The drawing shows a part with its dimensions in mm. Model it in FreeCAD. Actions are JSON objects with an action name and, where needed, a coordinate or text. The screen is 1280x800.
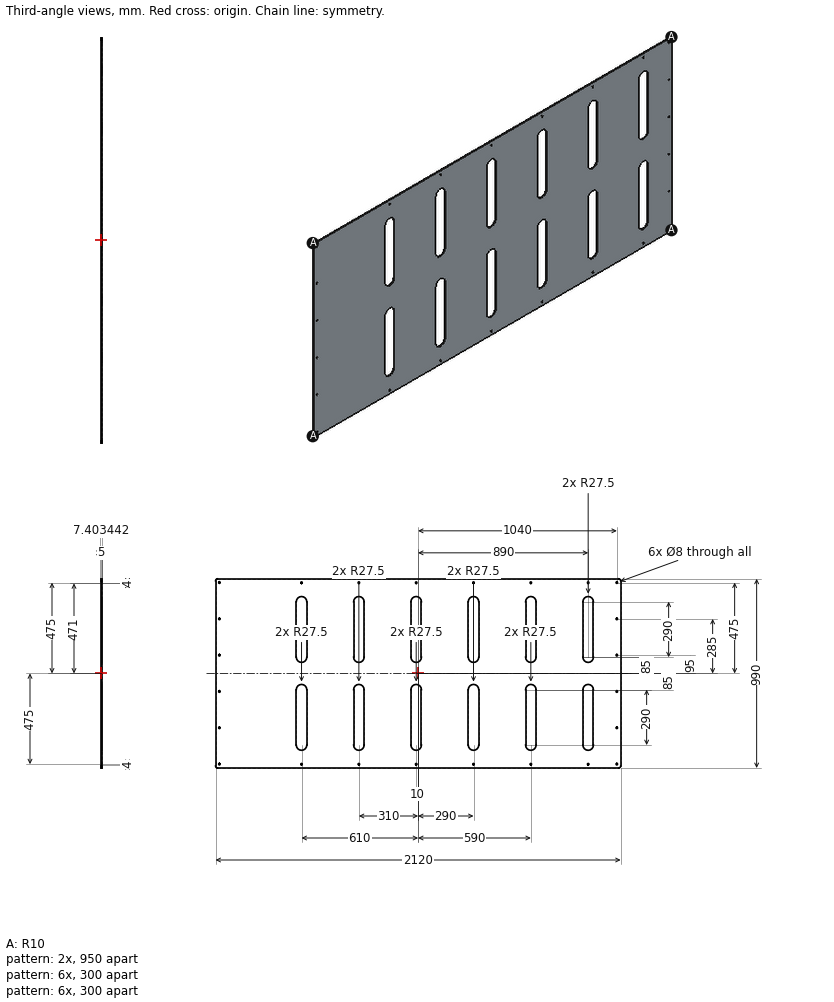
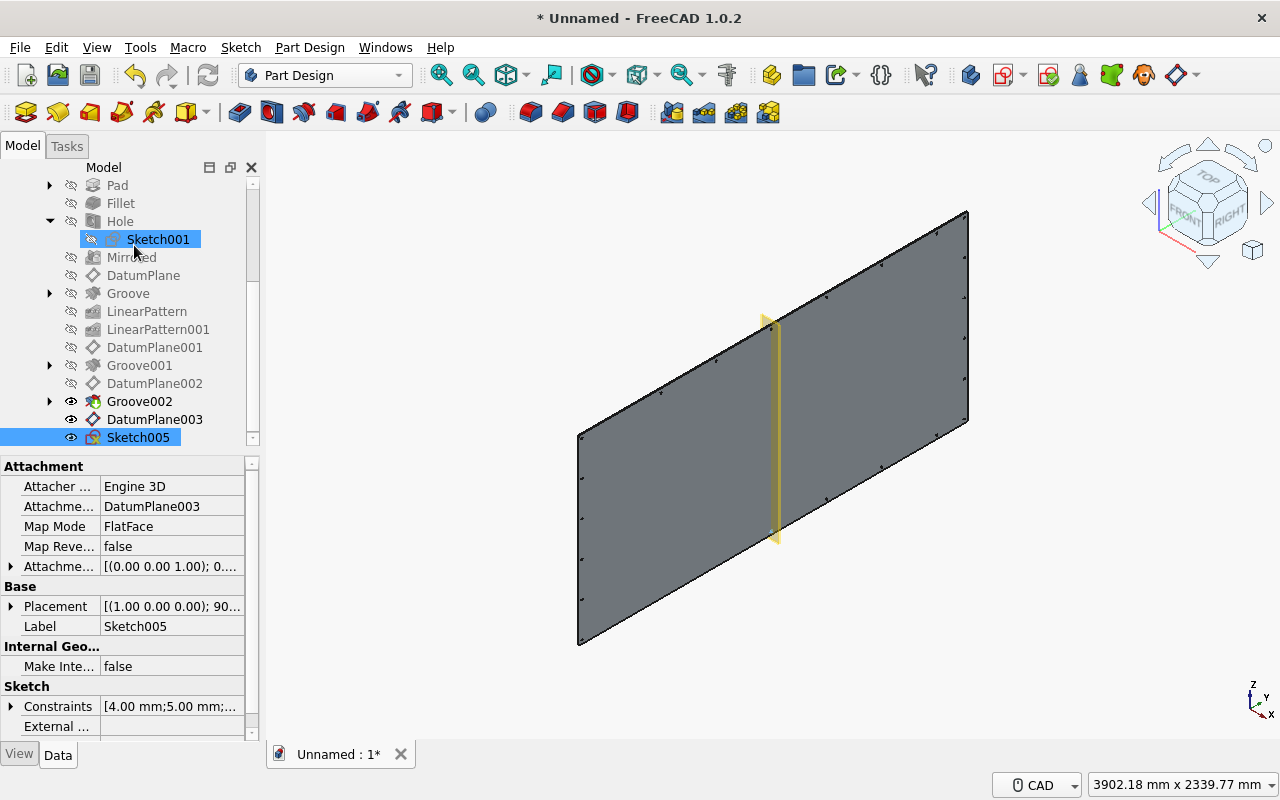
{"action": "left_click", "coordinate": [304, 112]}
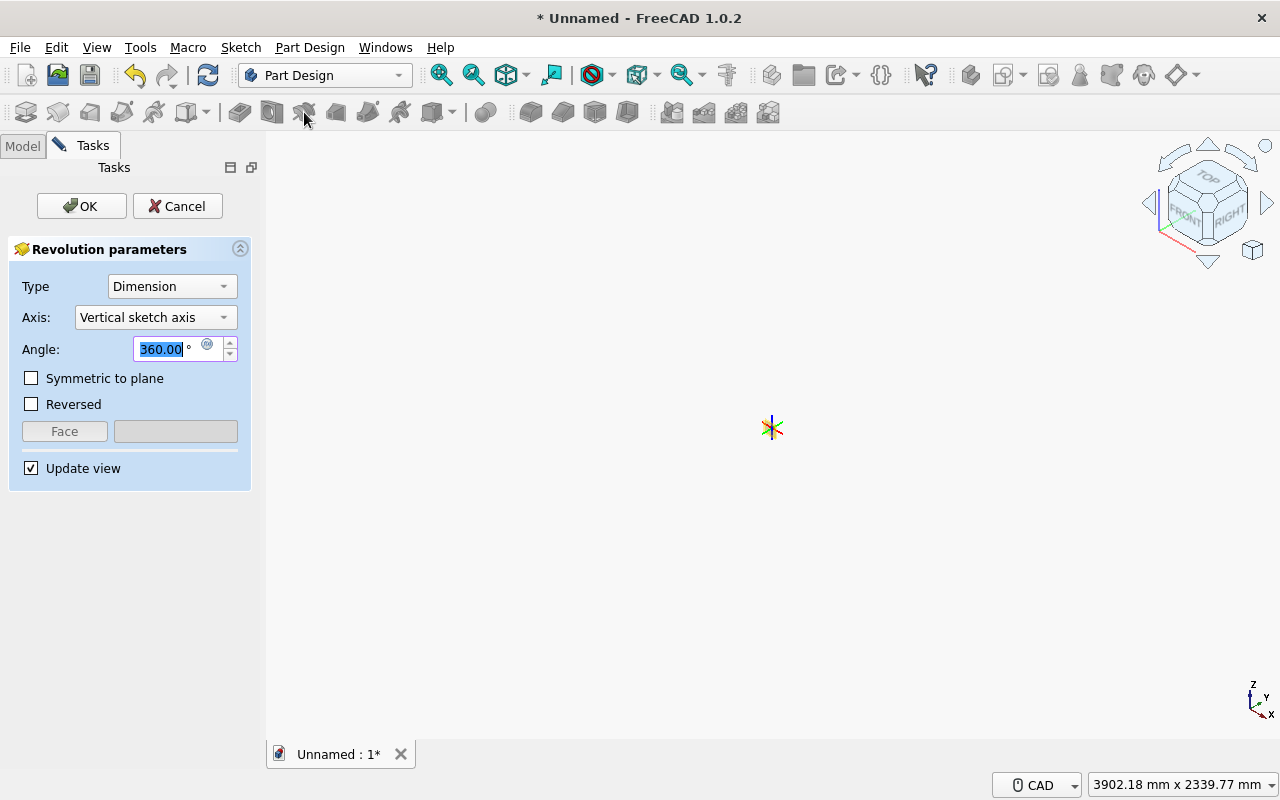
{"action": "left_click", "coordinate": [156, 318]}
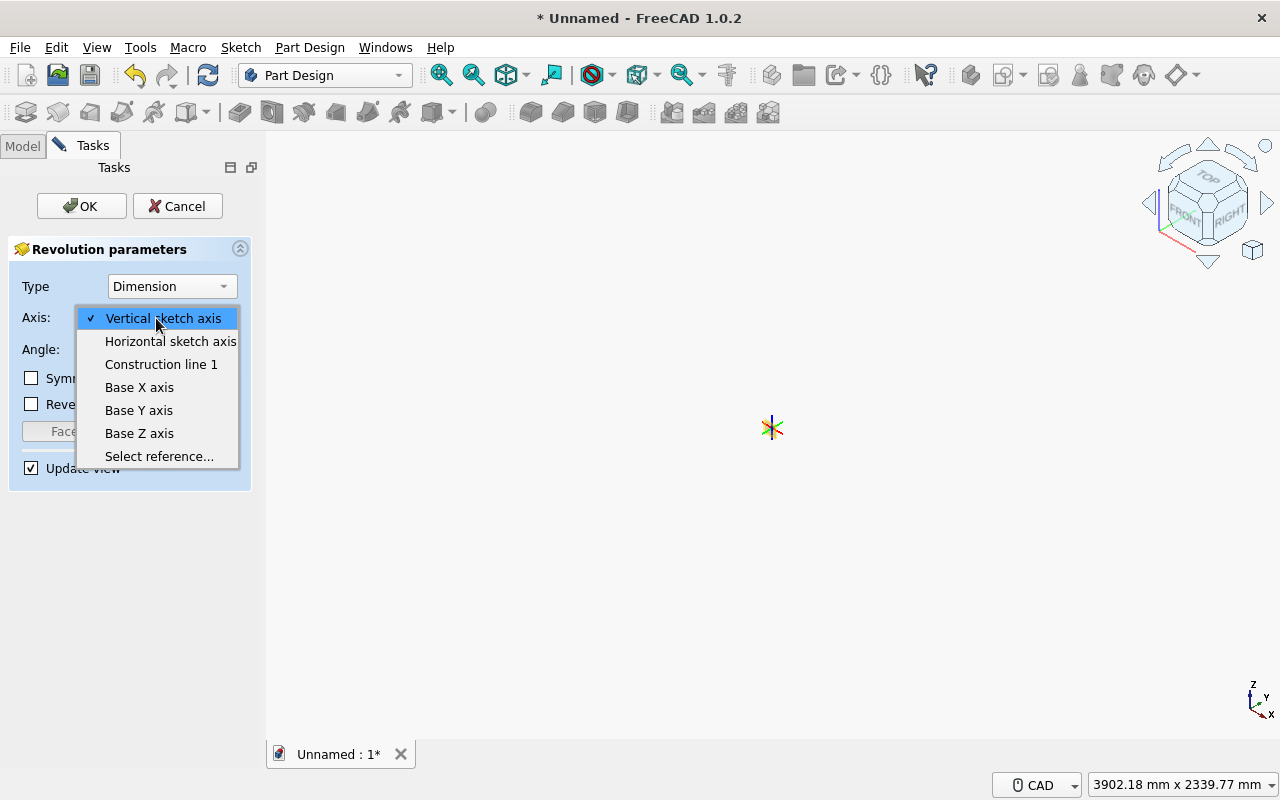
{"action": "left_click", "coordinate": [156, 364]}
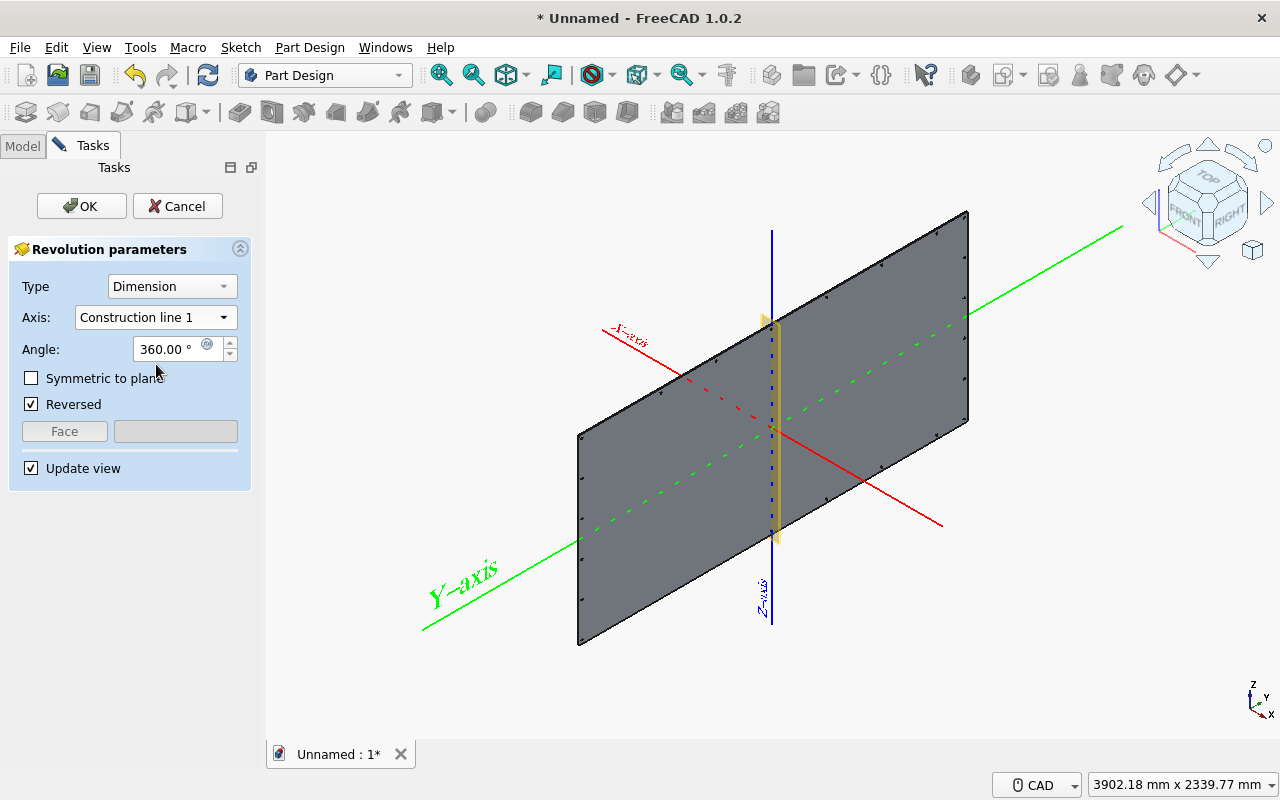
{"action": "left_click", "coordinate": [82, 206]}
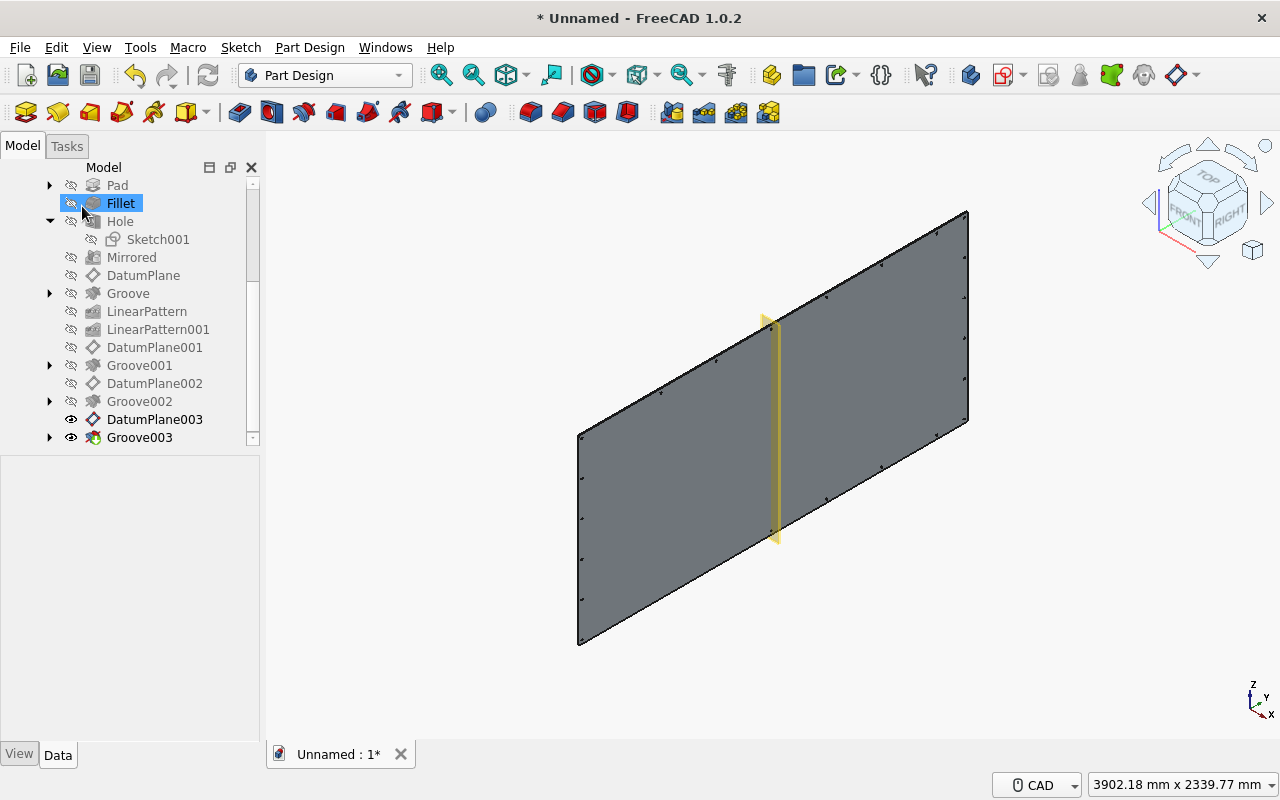
{"action": "left_click", "coordinate": [116, 419]}
{"action": "key", "text": "space"}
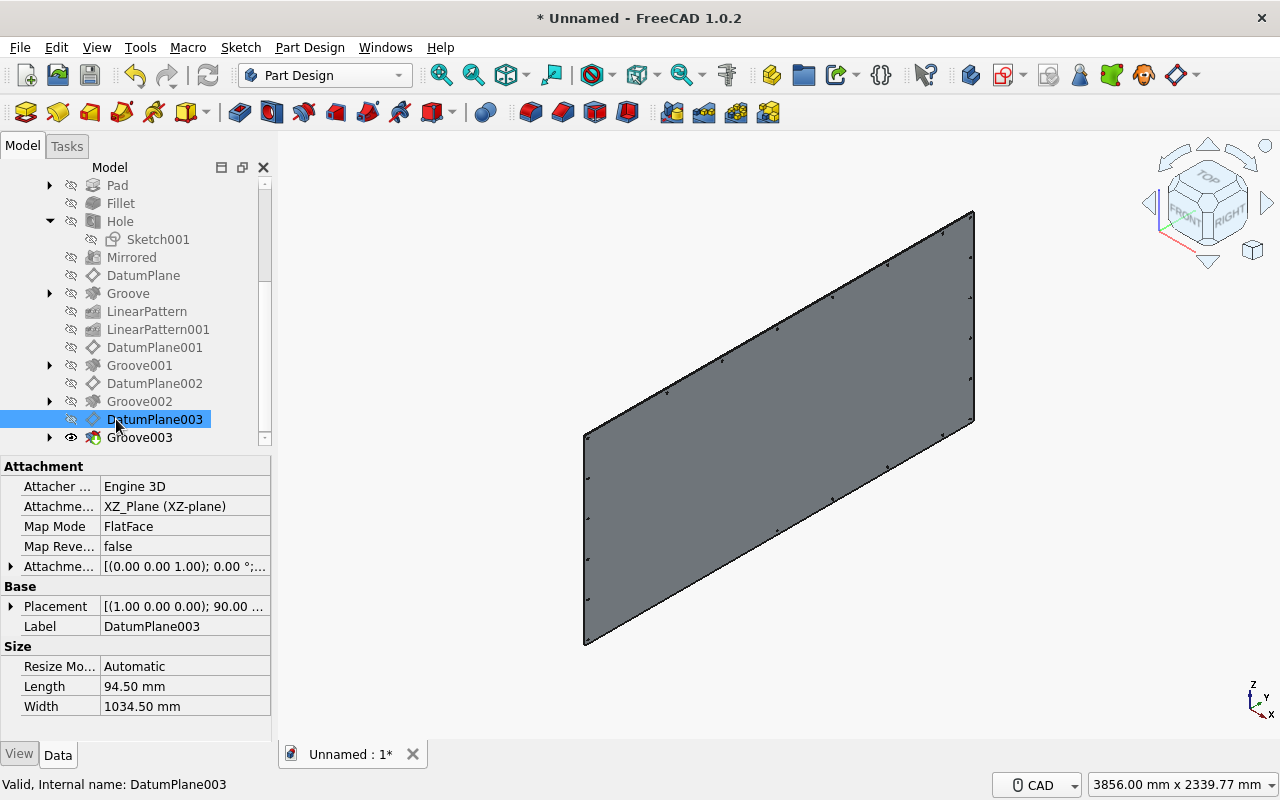
{"action": "scroll", "coordinate": [140, 307], "scroll_direction": "down", "scroll_amount": 3}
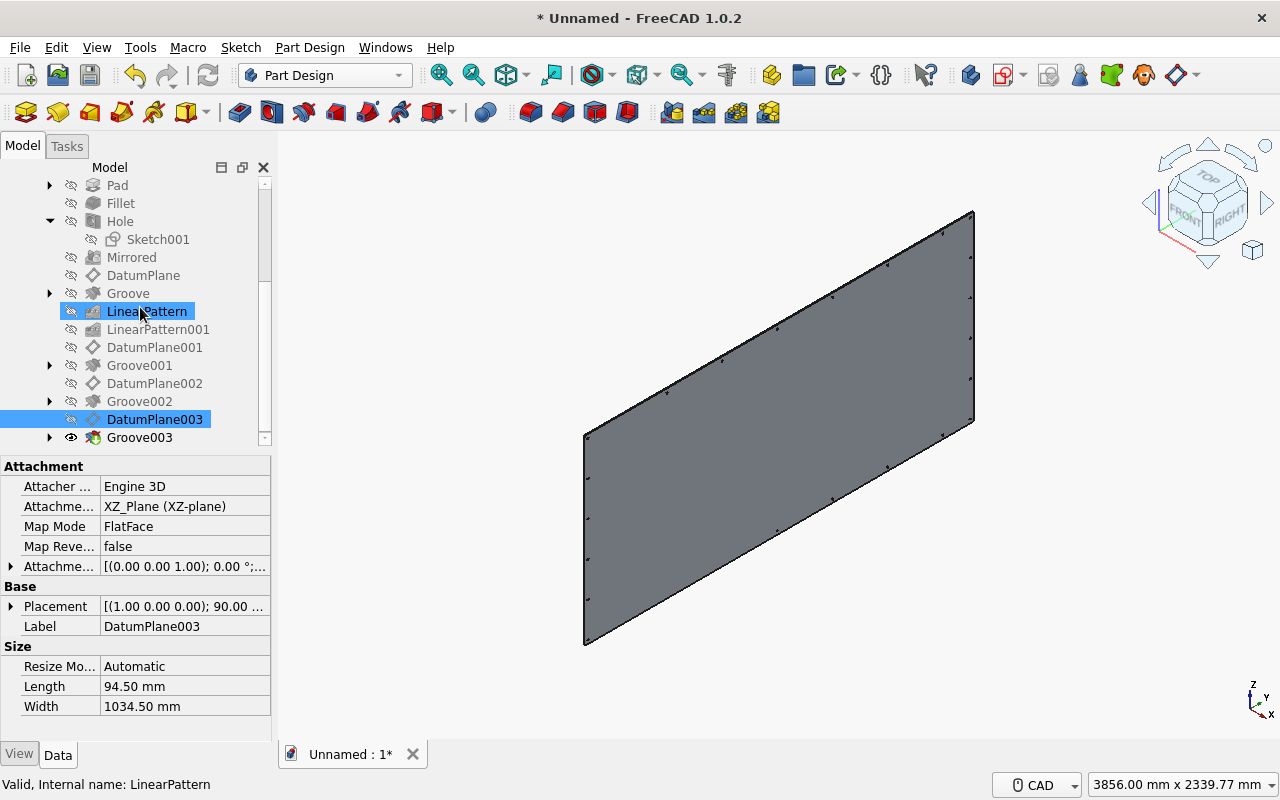
{"action": "scroll", "coordinate": [140, 307], "scroll_direction": "up", "scroll_amount": 15}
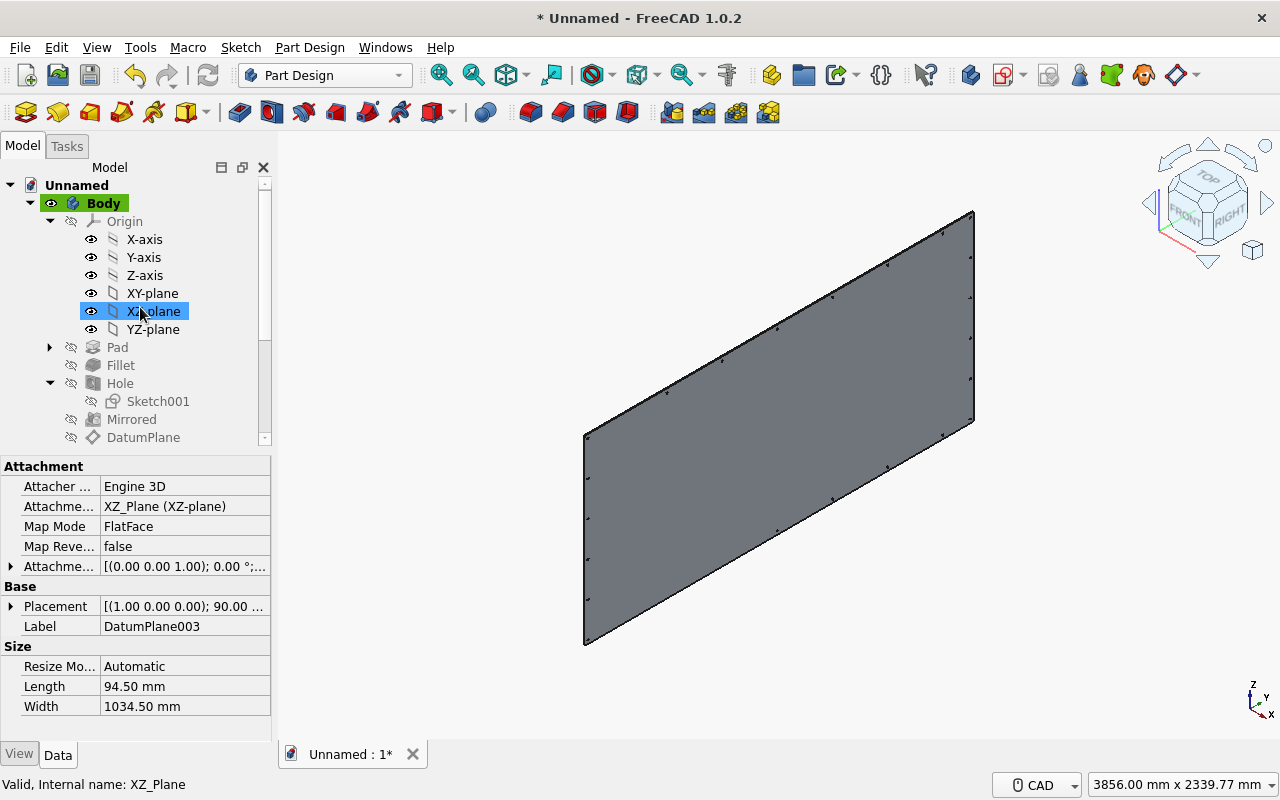
{"action": "left_click", "coordinate": [136, 311]}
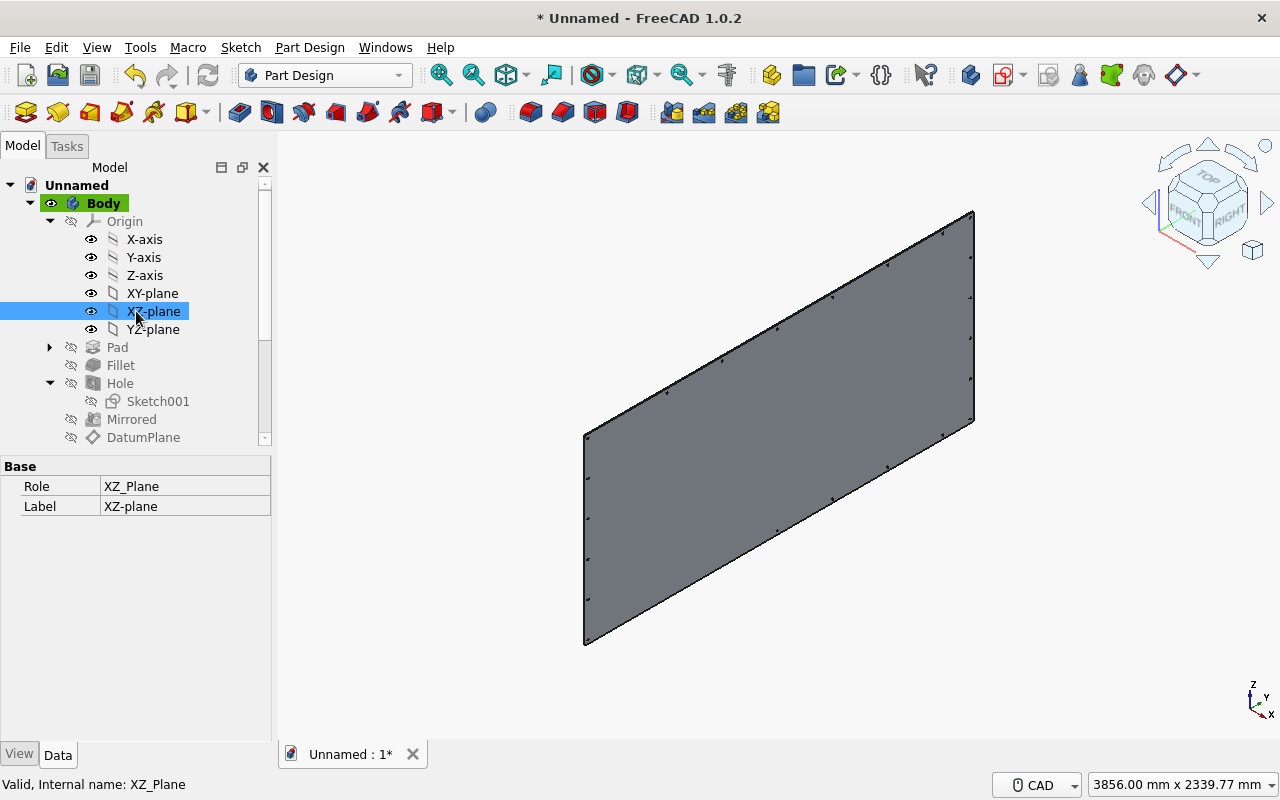
{"action": "left_click", "coordinate": [1176, 76]}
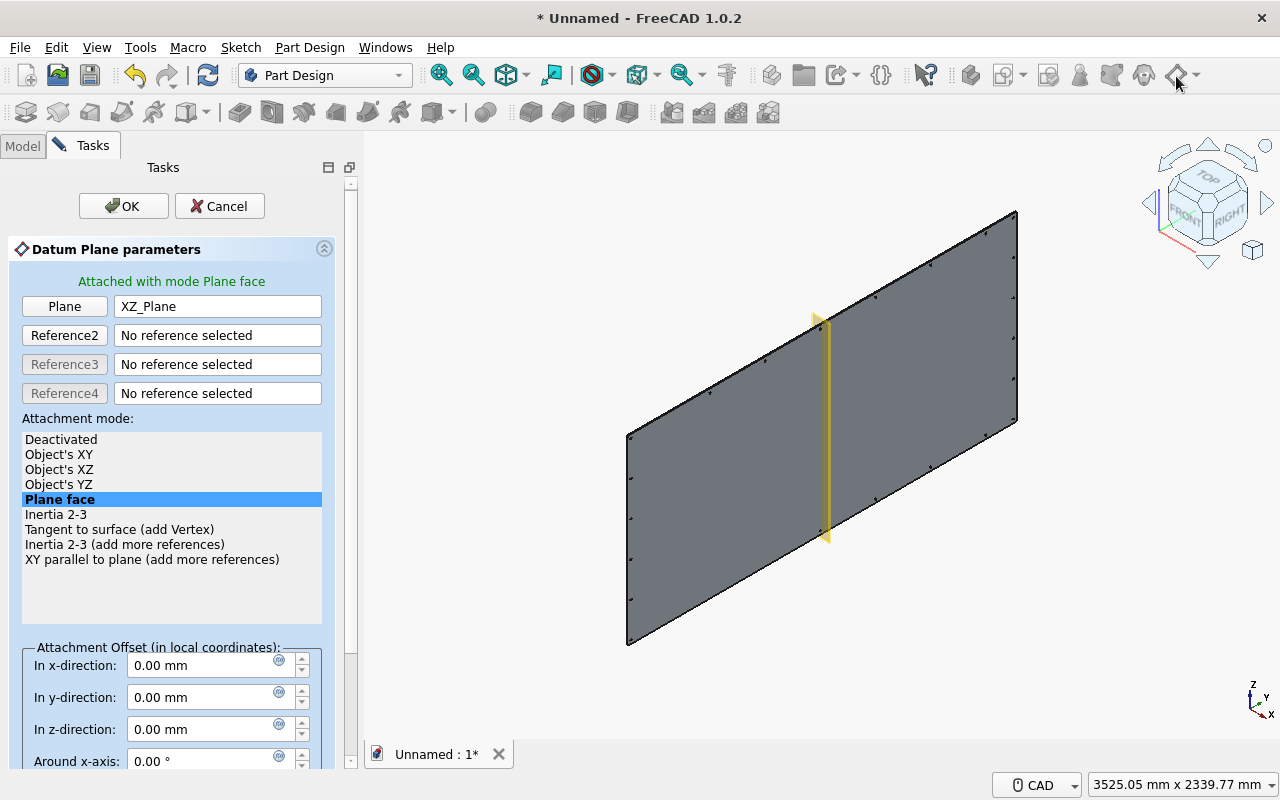
{"action": "triple_click", "coordinate": [210, 729]}